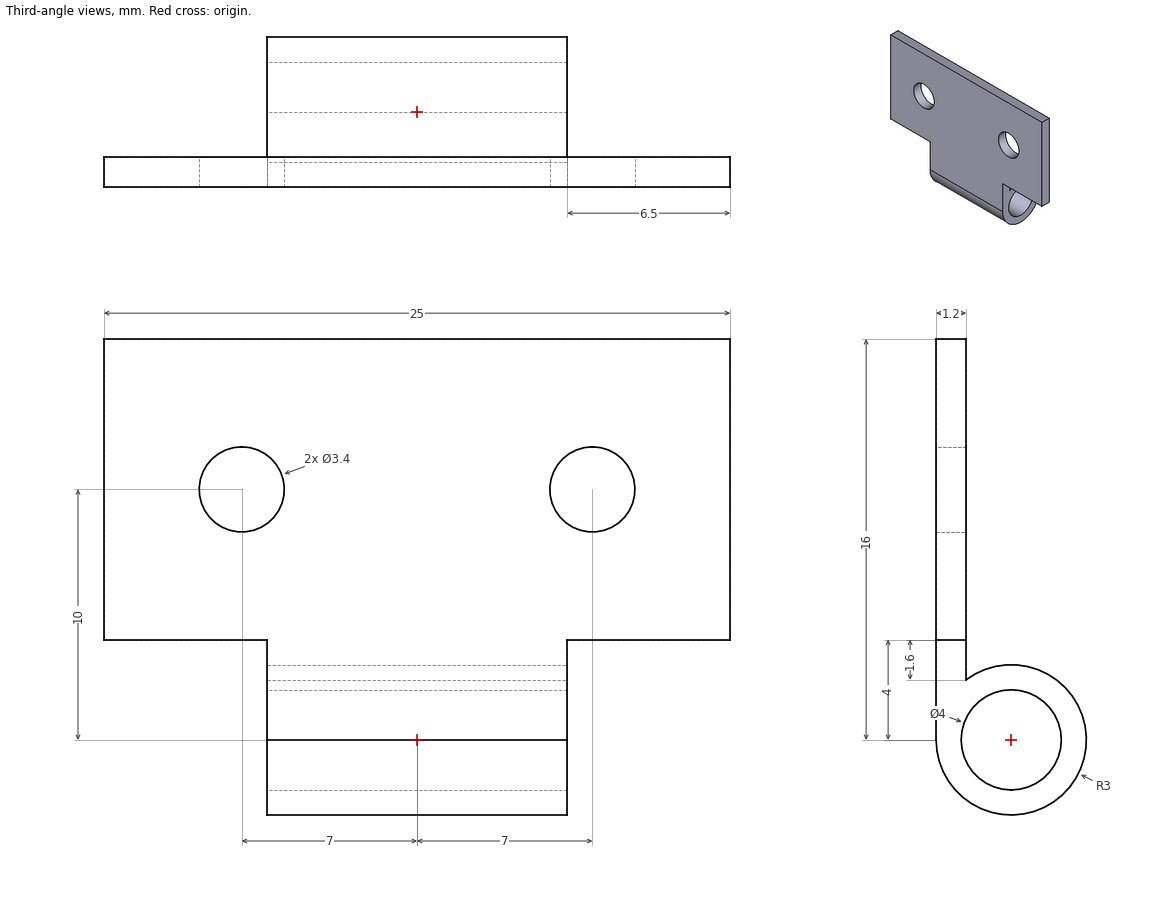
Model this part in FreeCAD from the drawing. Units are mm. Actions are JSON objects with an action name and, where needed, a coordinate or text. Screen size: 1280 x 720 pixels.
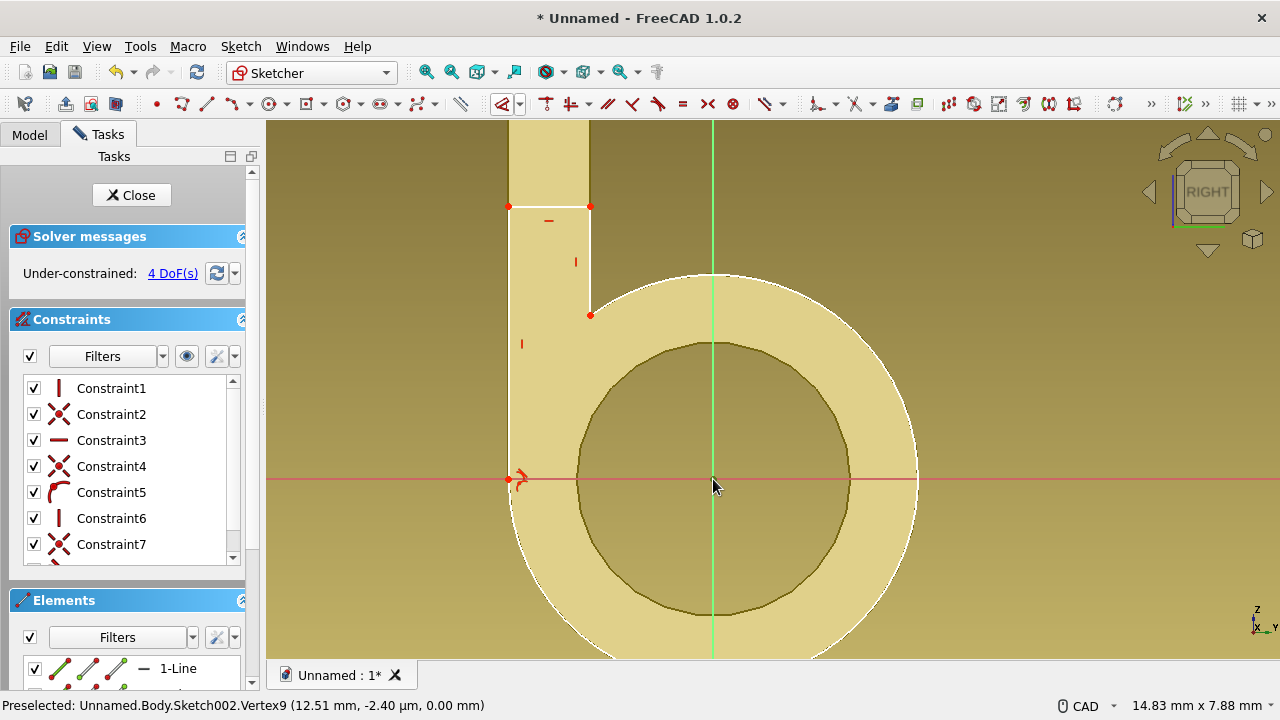
{"action": "left_click", "coordinate": [714, 596]}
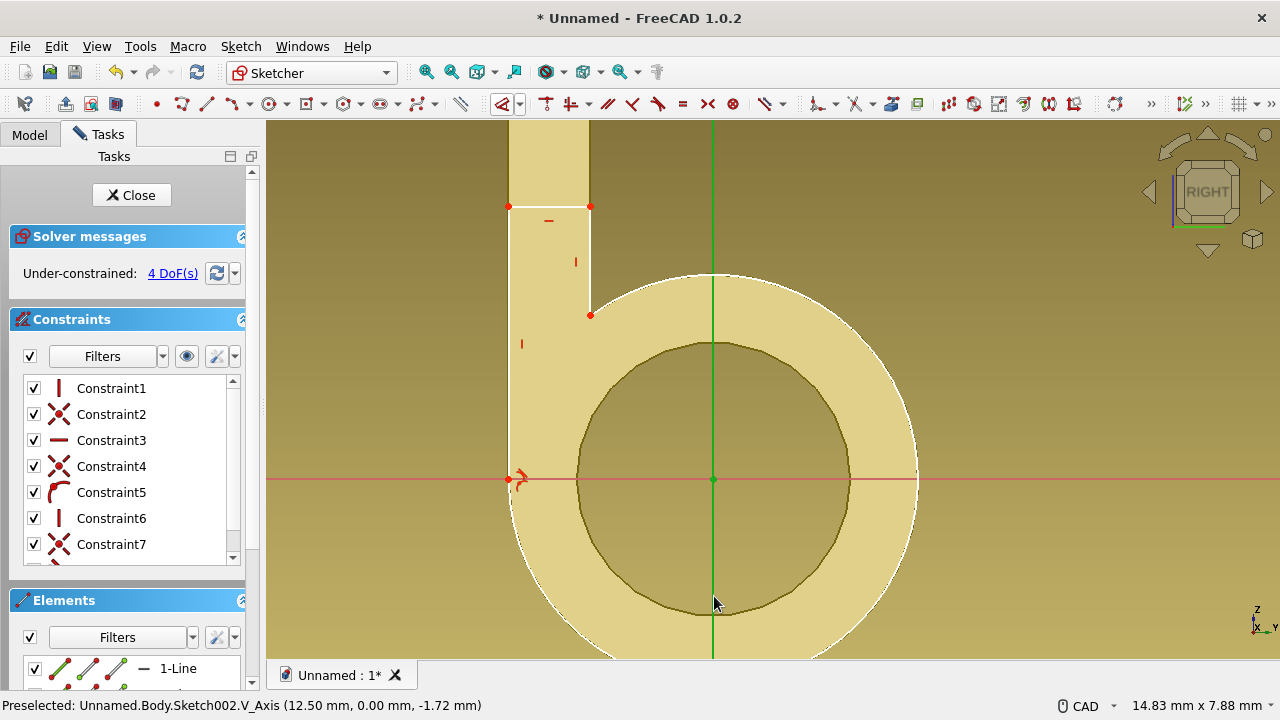
{"action": "left_click", "coordinate": [546, 104]}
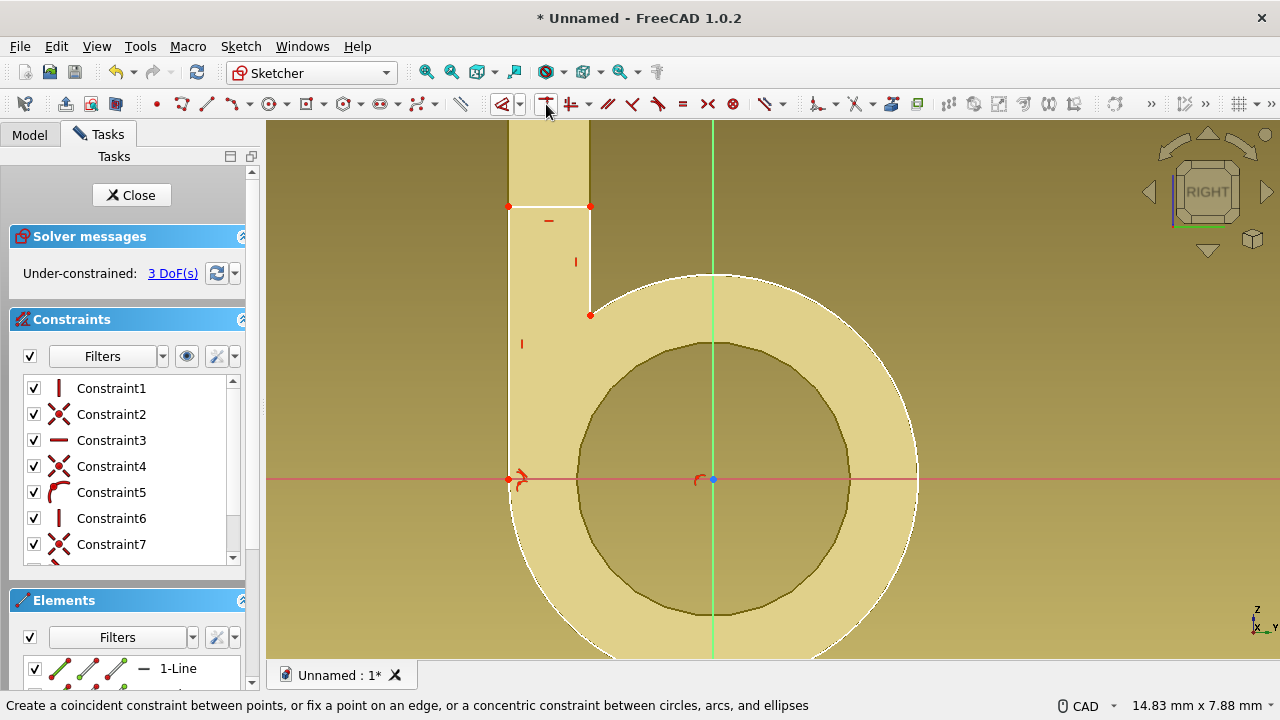
{"action": "left_click", "coordinate": [881, 362]}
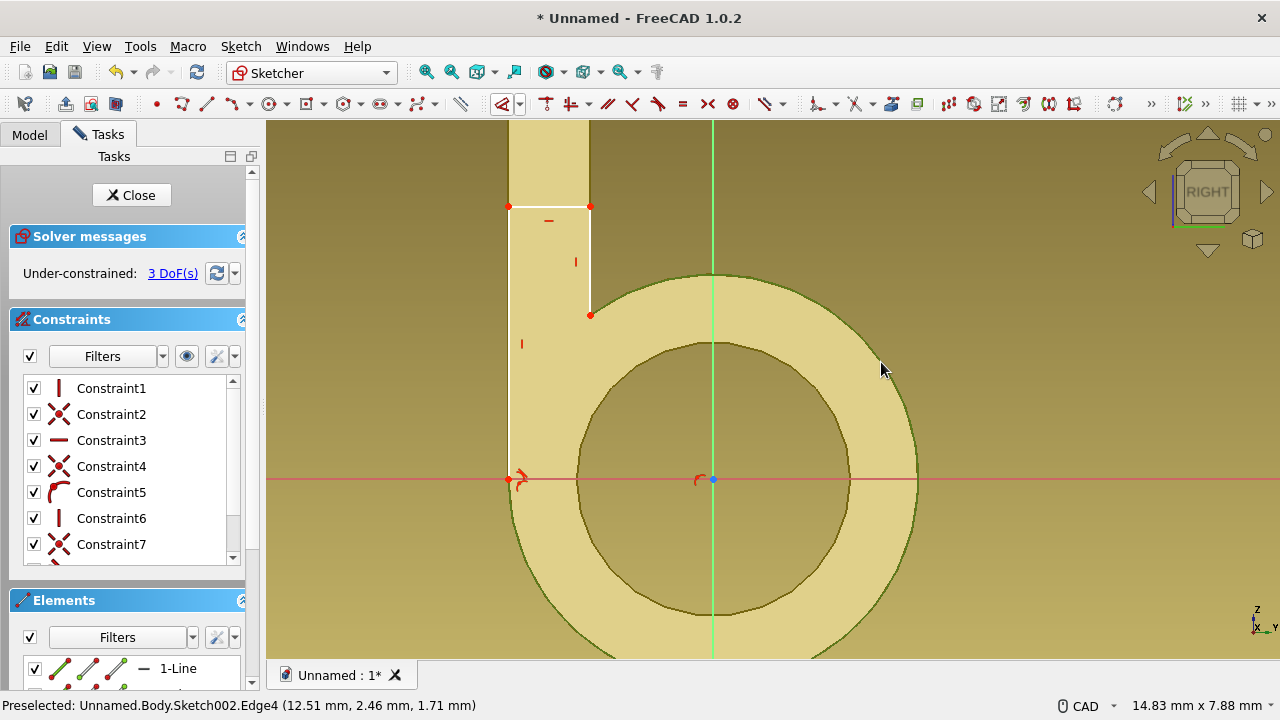
{"action": "left_click", "coordinate": [520, 104]}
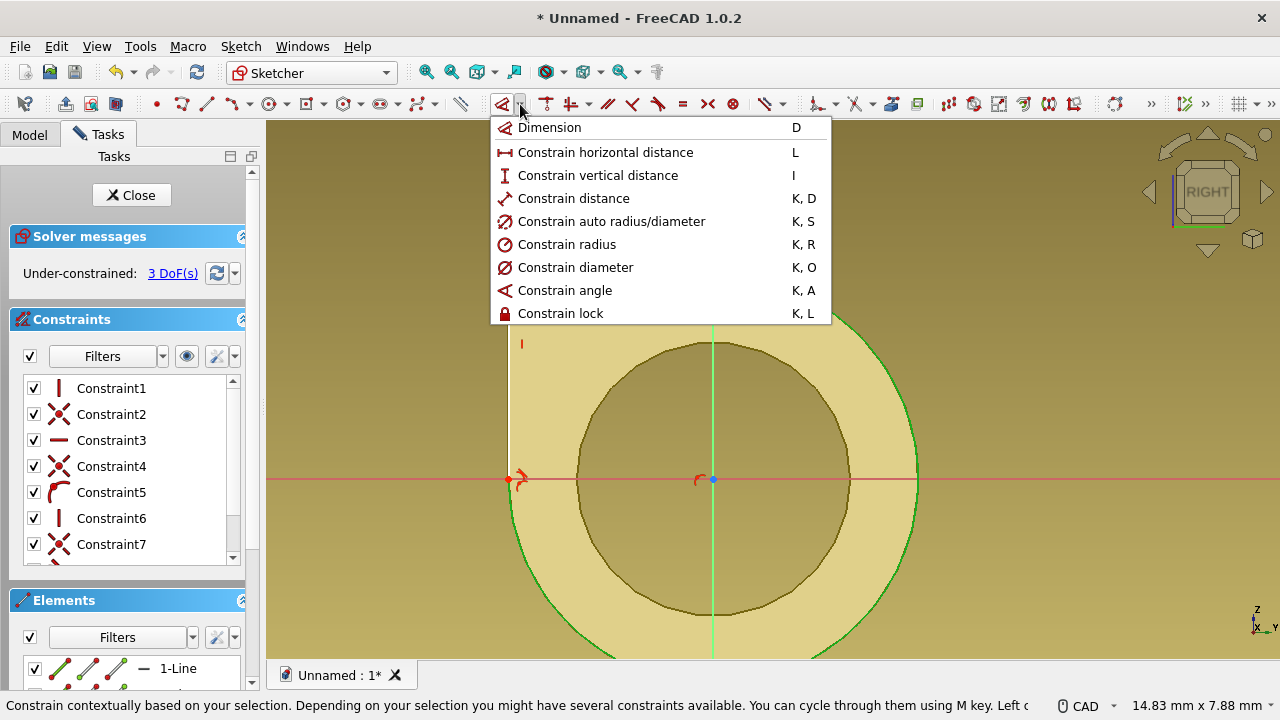
{"action": "left_click", "coordinate": [661, 244]}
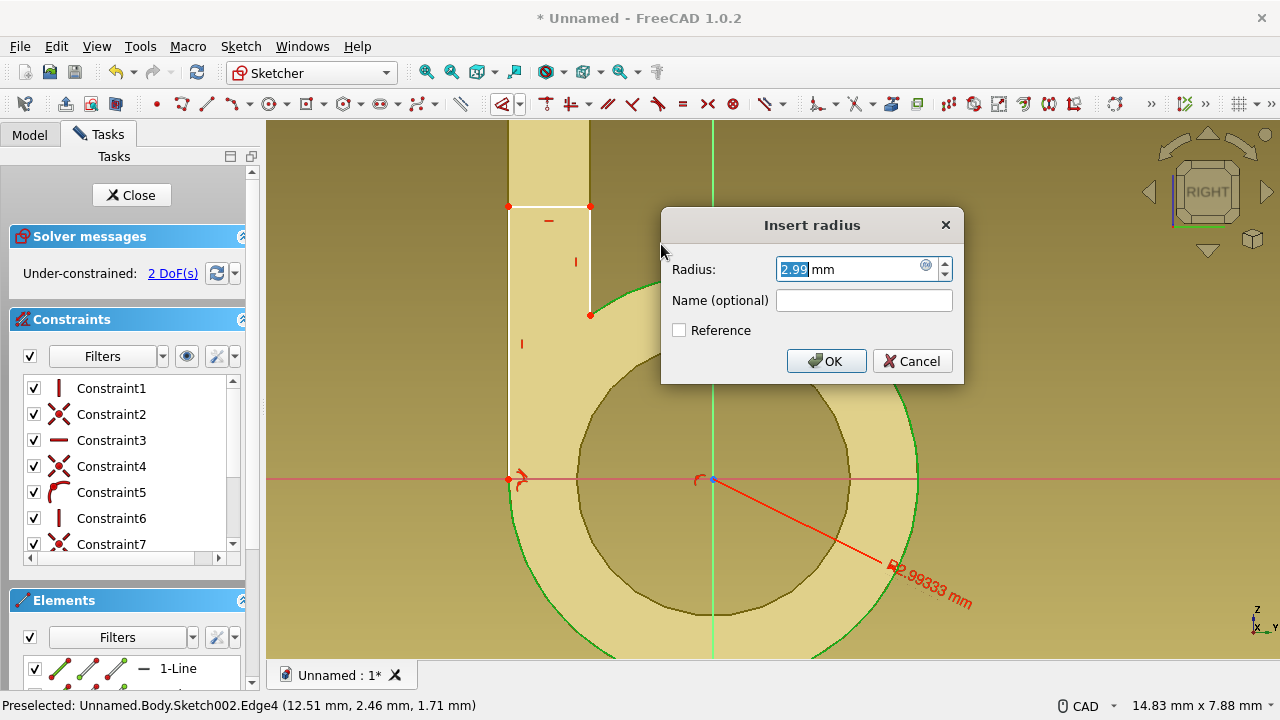
{"action": "type", "text": "3"}
{"action": "key", "text": "Return"}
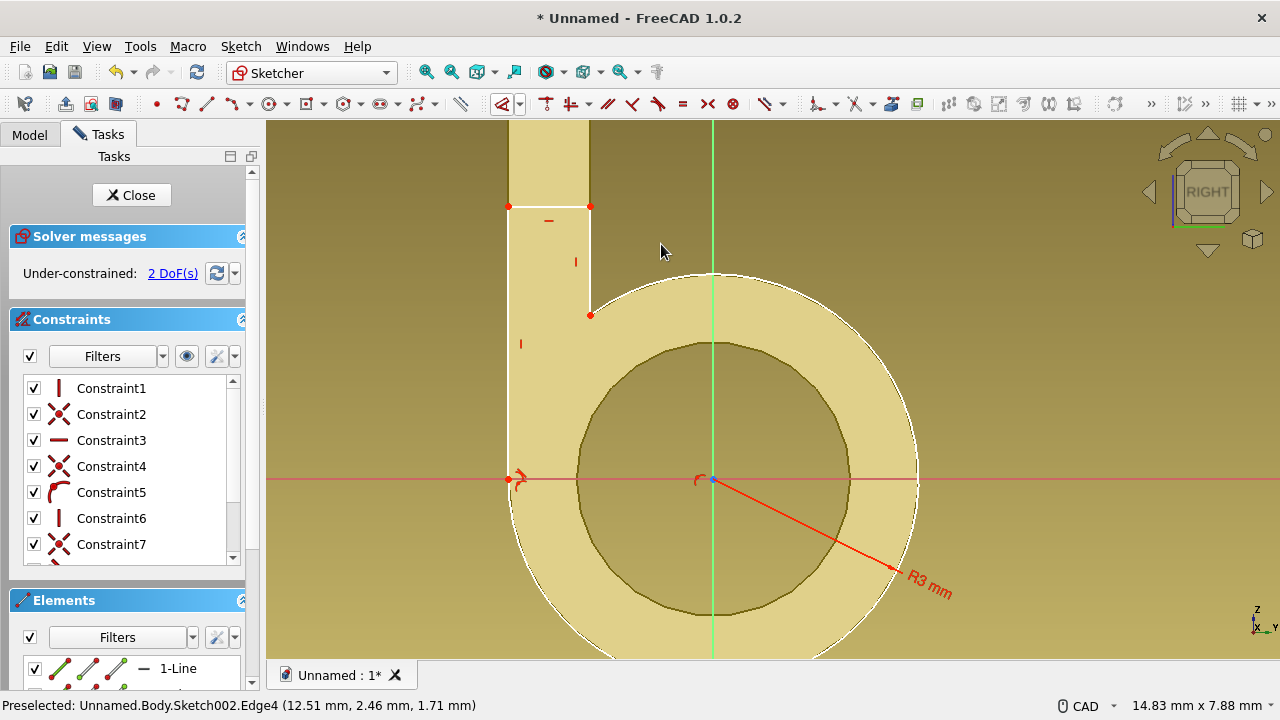
{"action": "left_click", "coordinate": [508, 289]}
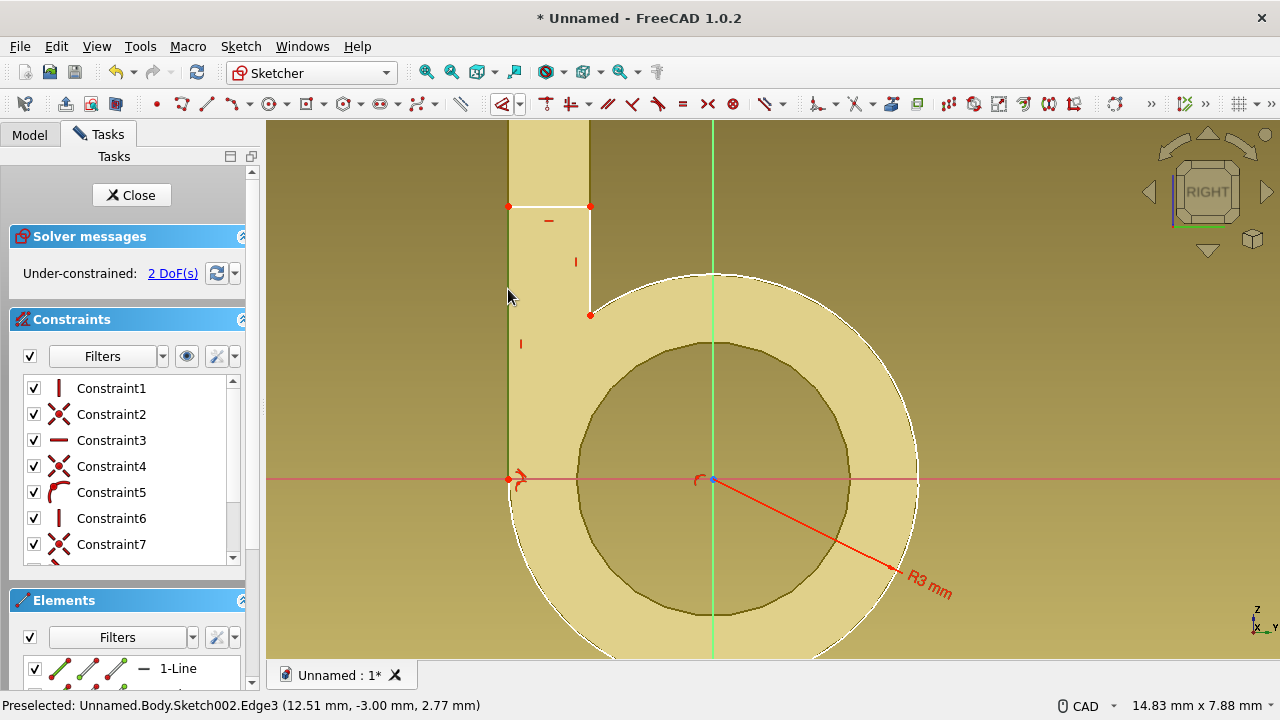
{"action": "key", "text": "i"}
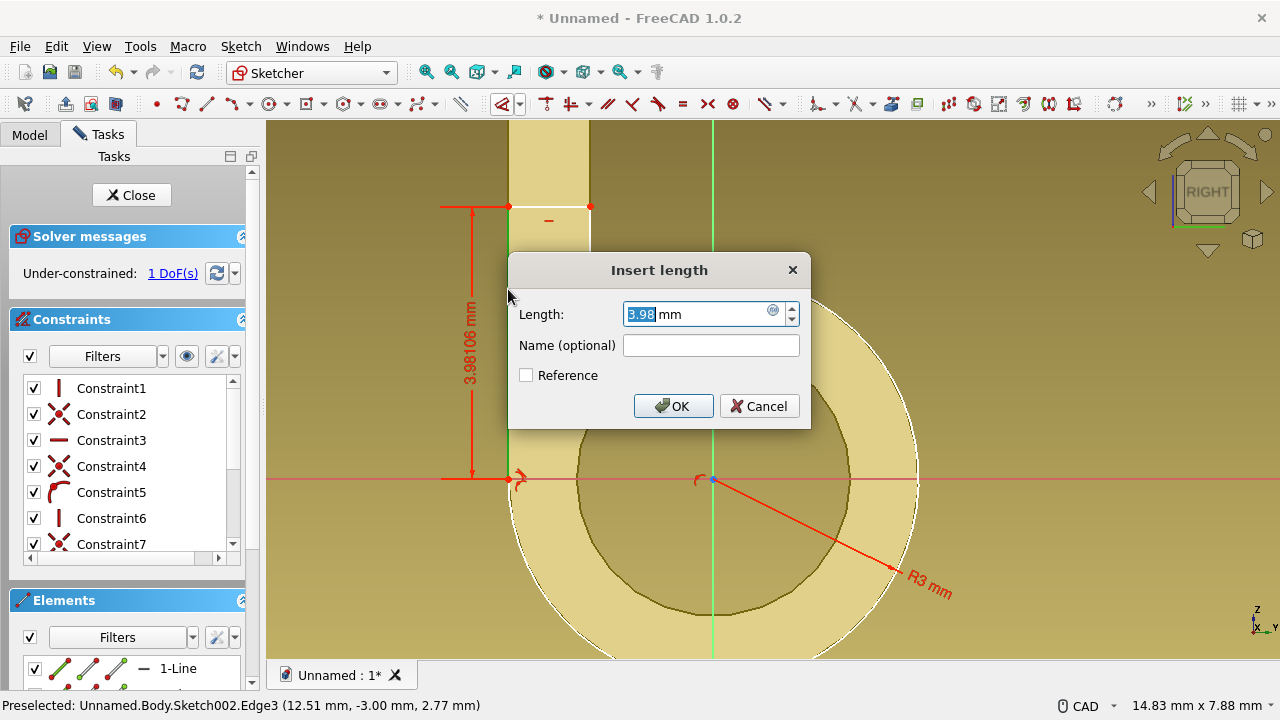
{"action": "type", "text": "4"}
{"action": "key", "text": "Return"}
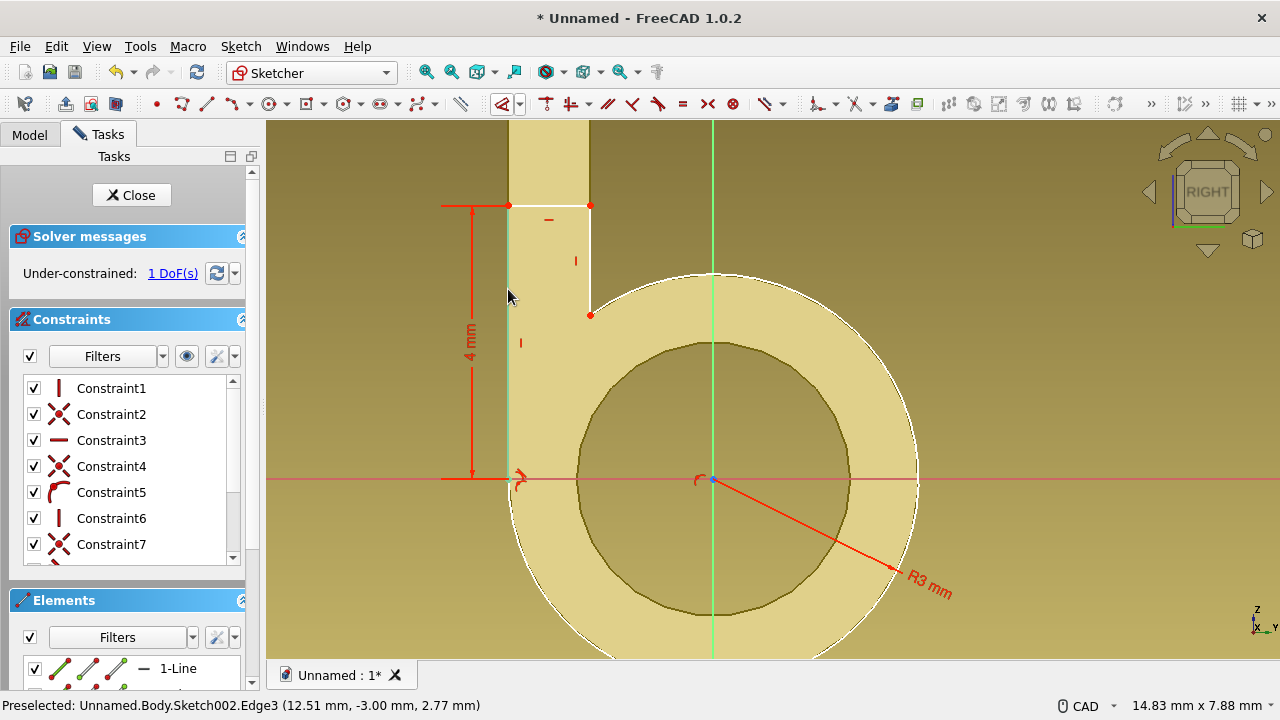
{"action": "left_click", "coordinate": [590, 283]}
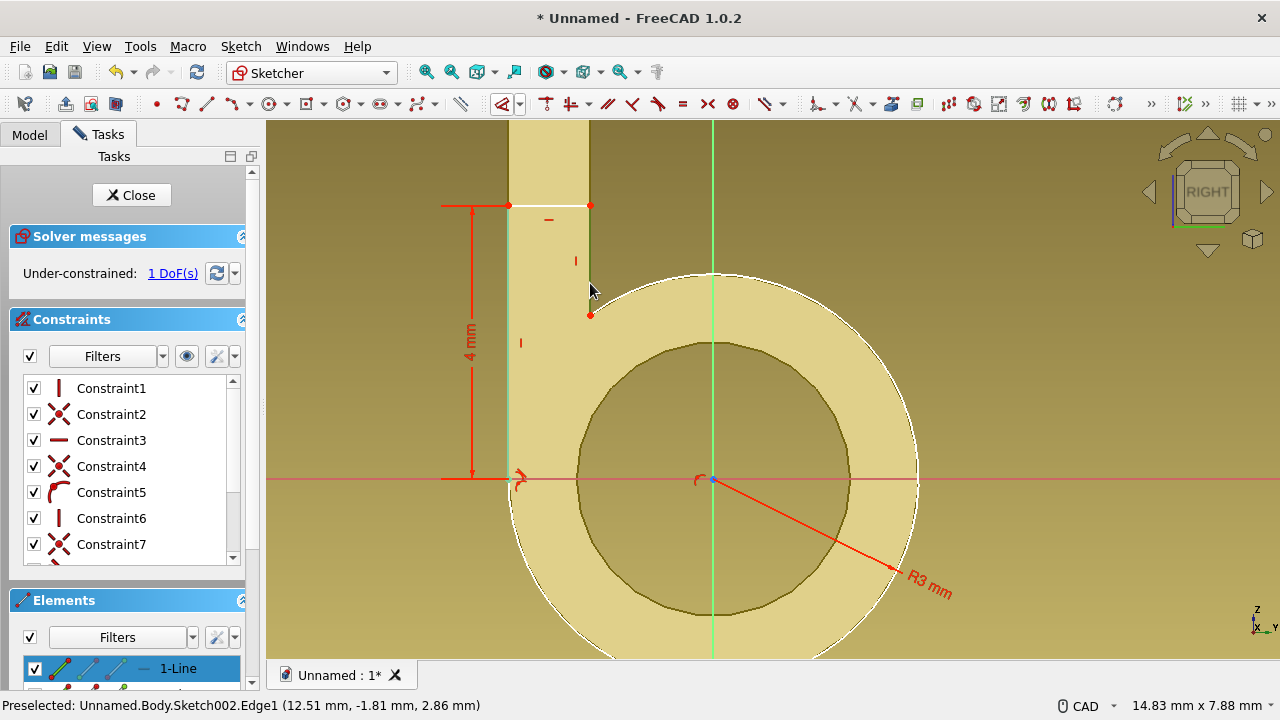
{"action": "key", "text": "i"}